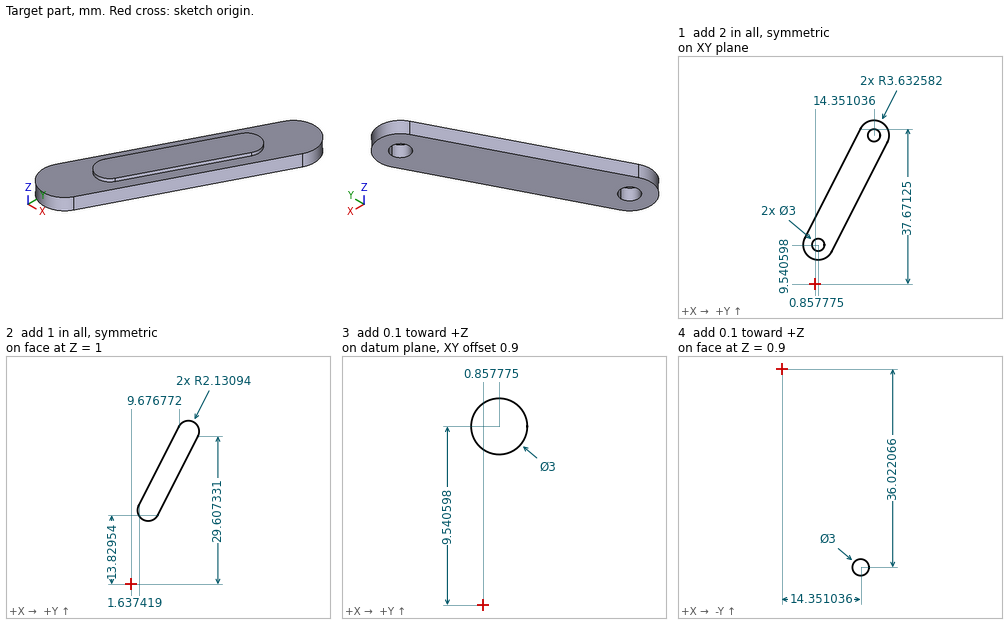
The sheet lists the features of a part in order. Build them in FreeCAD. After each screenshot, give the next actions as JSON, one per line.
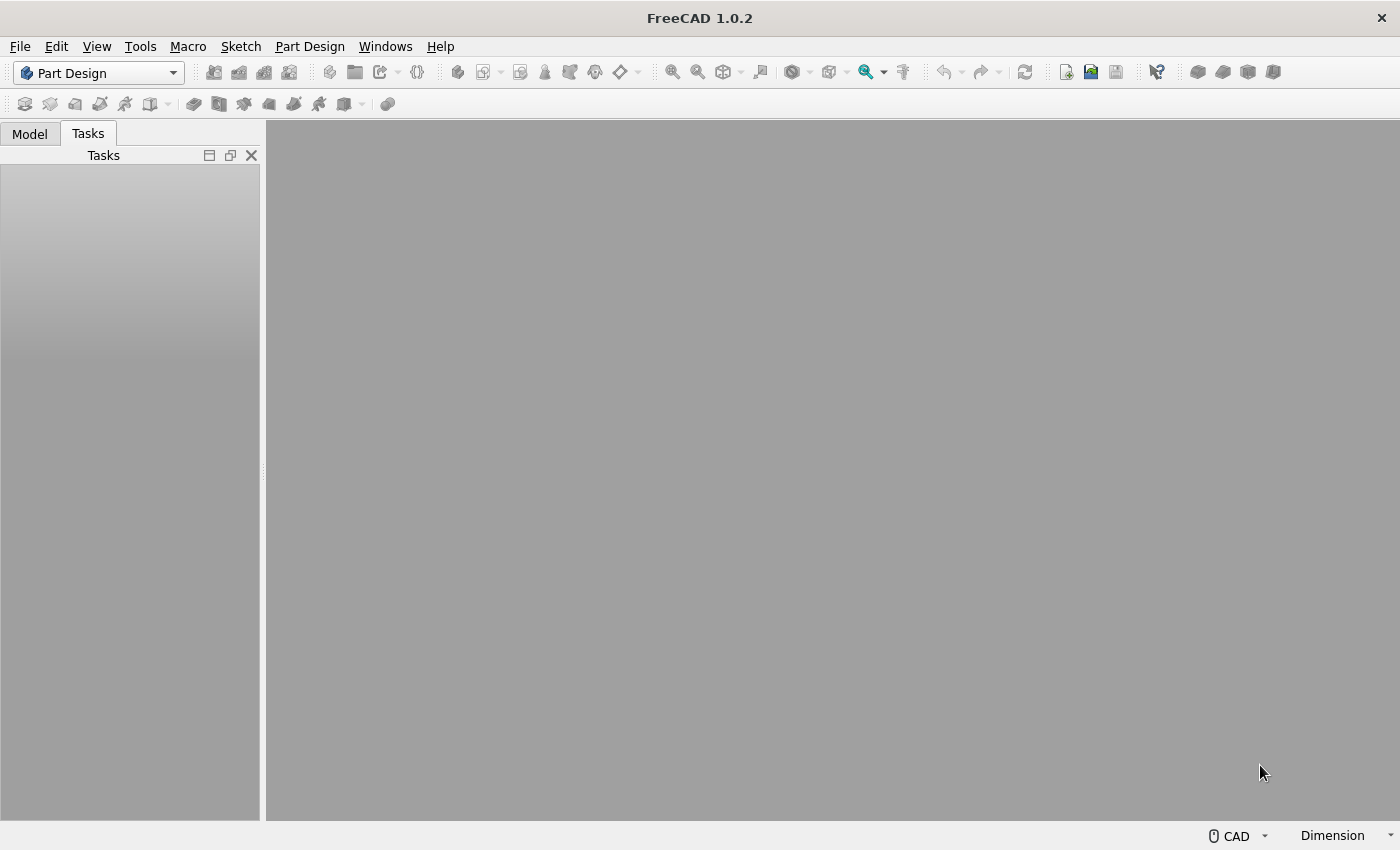
{"action": "left_click", "coordinate": [1066, 72]}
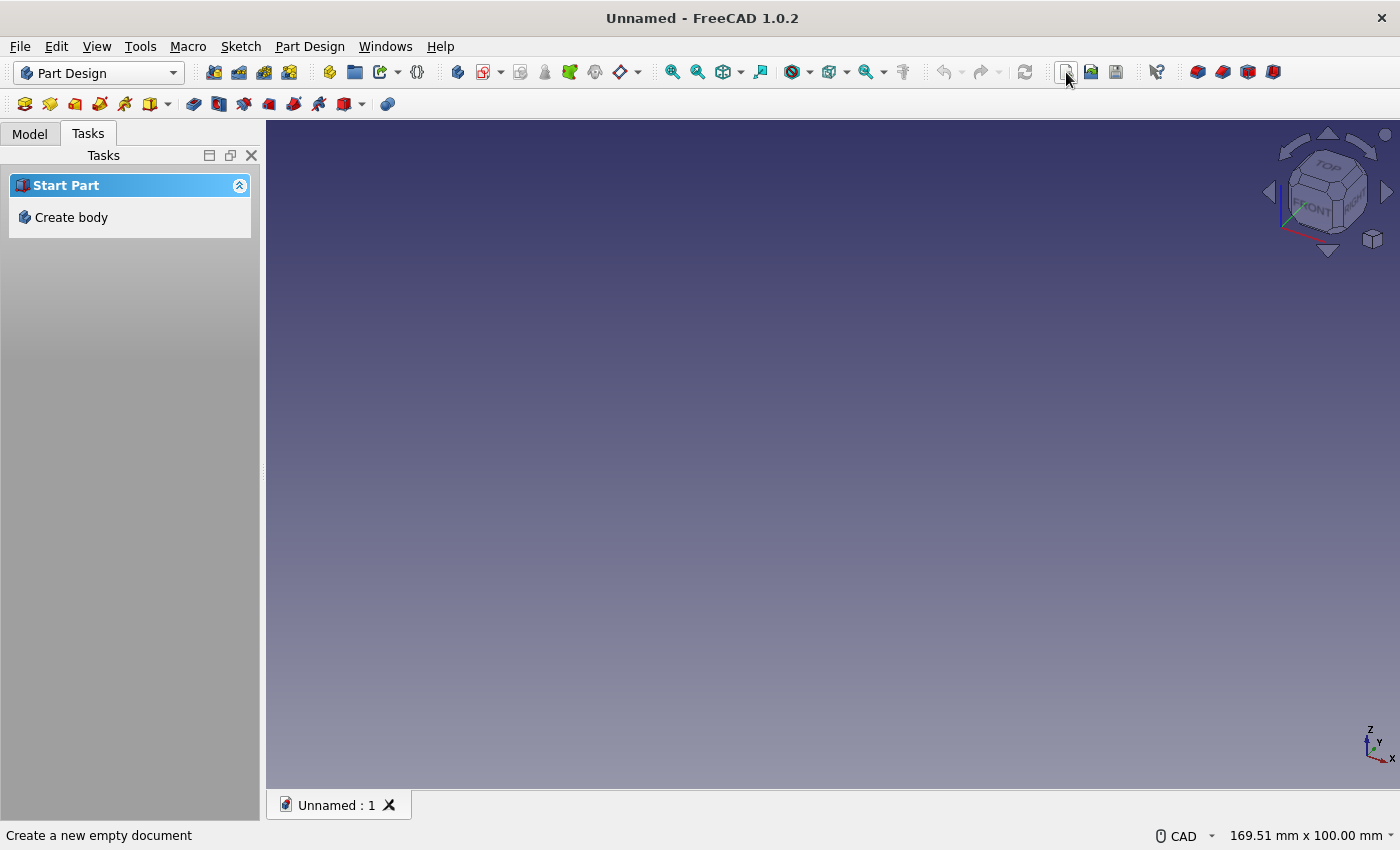
{"action": "left_click", "coordinate": [482, 72]}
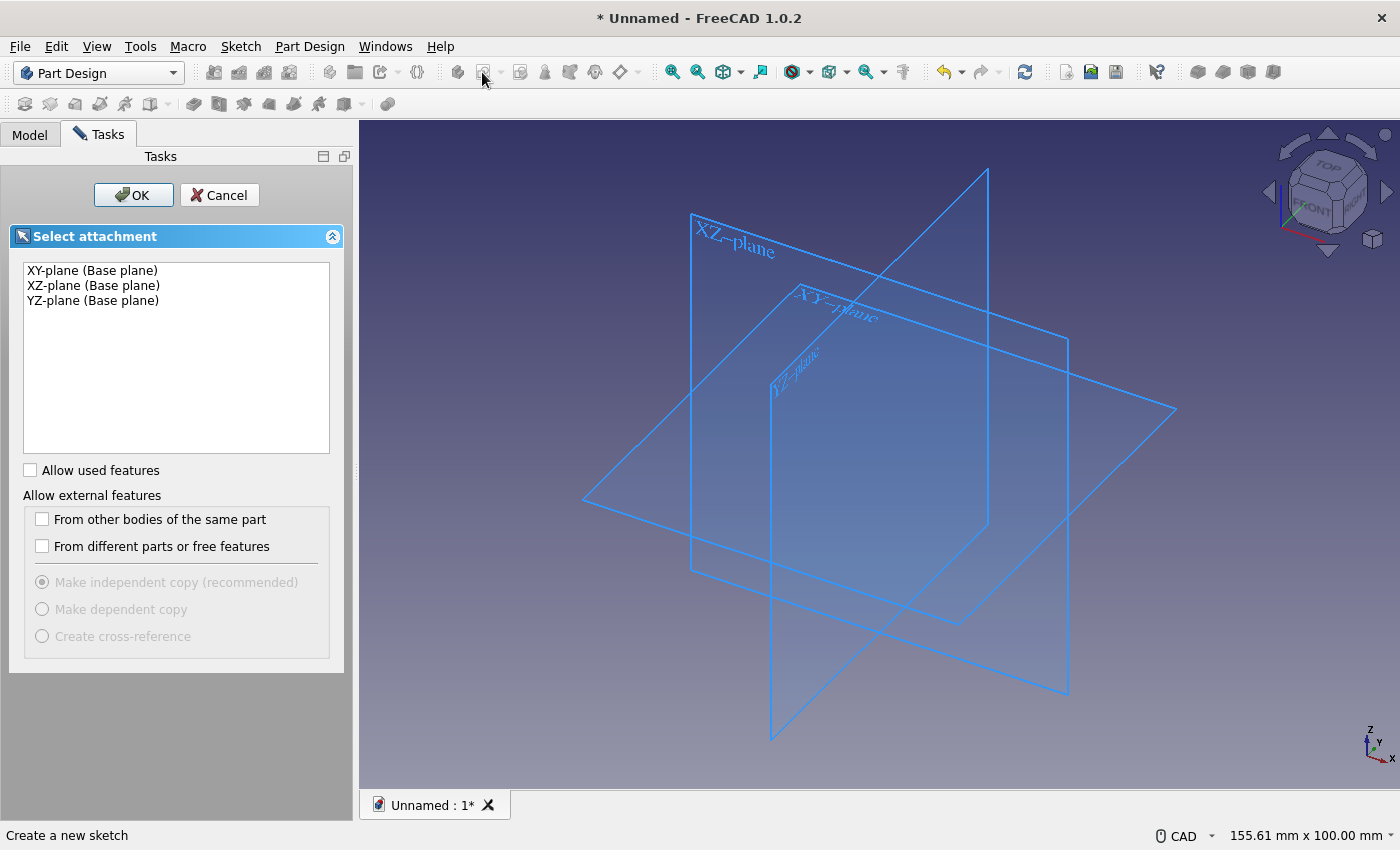
{"action": "left_click", "coordinate": [84, 270]}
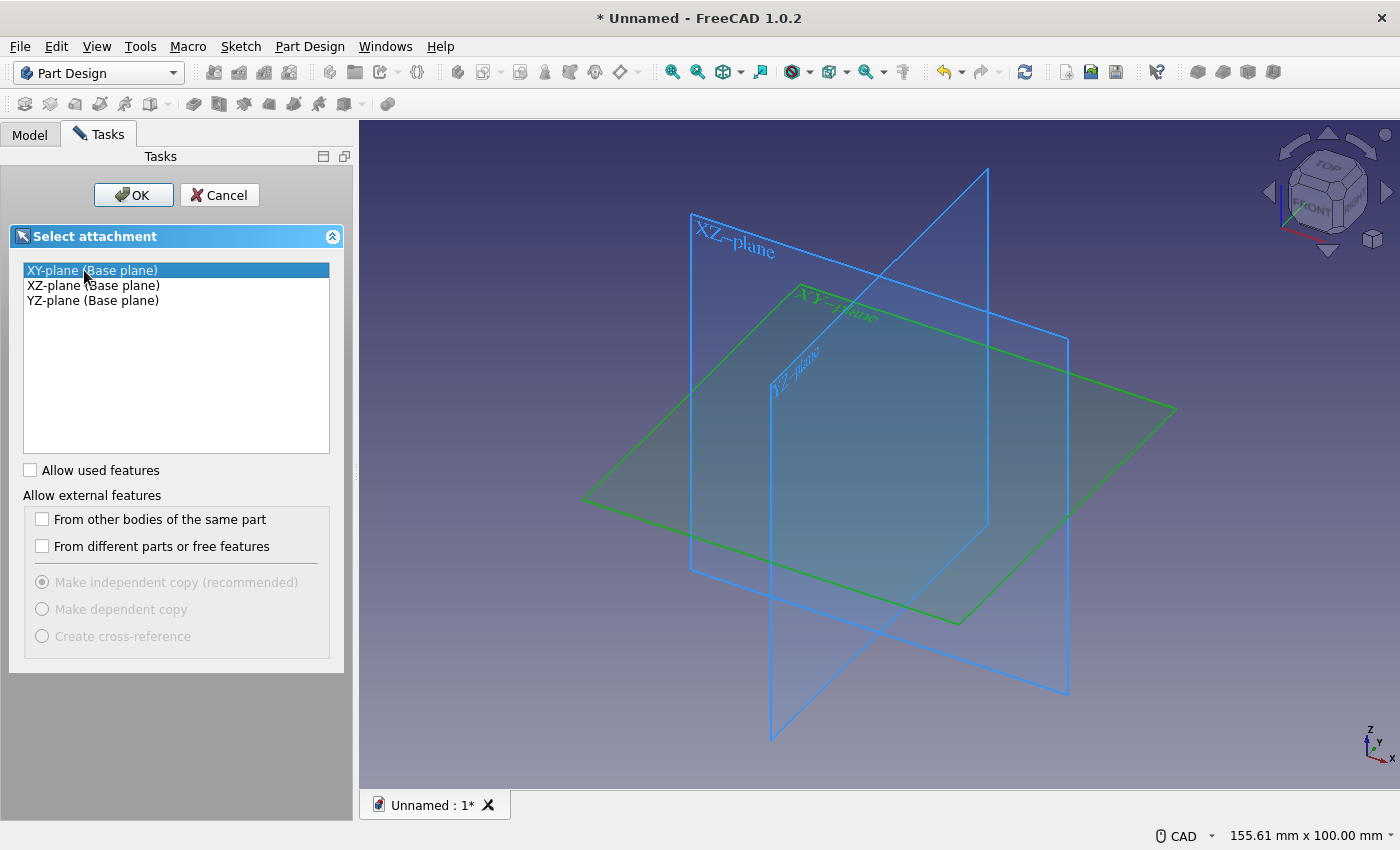
{"action": "left_click", "coordinate": [134, 195]}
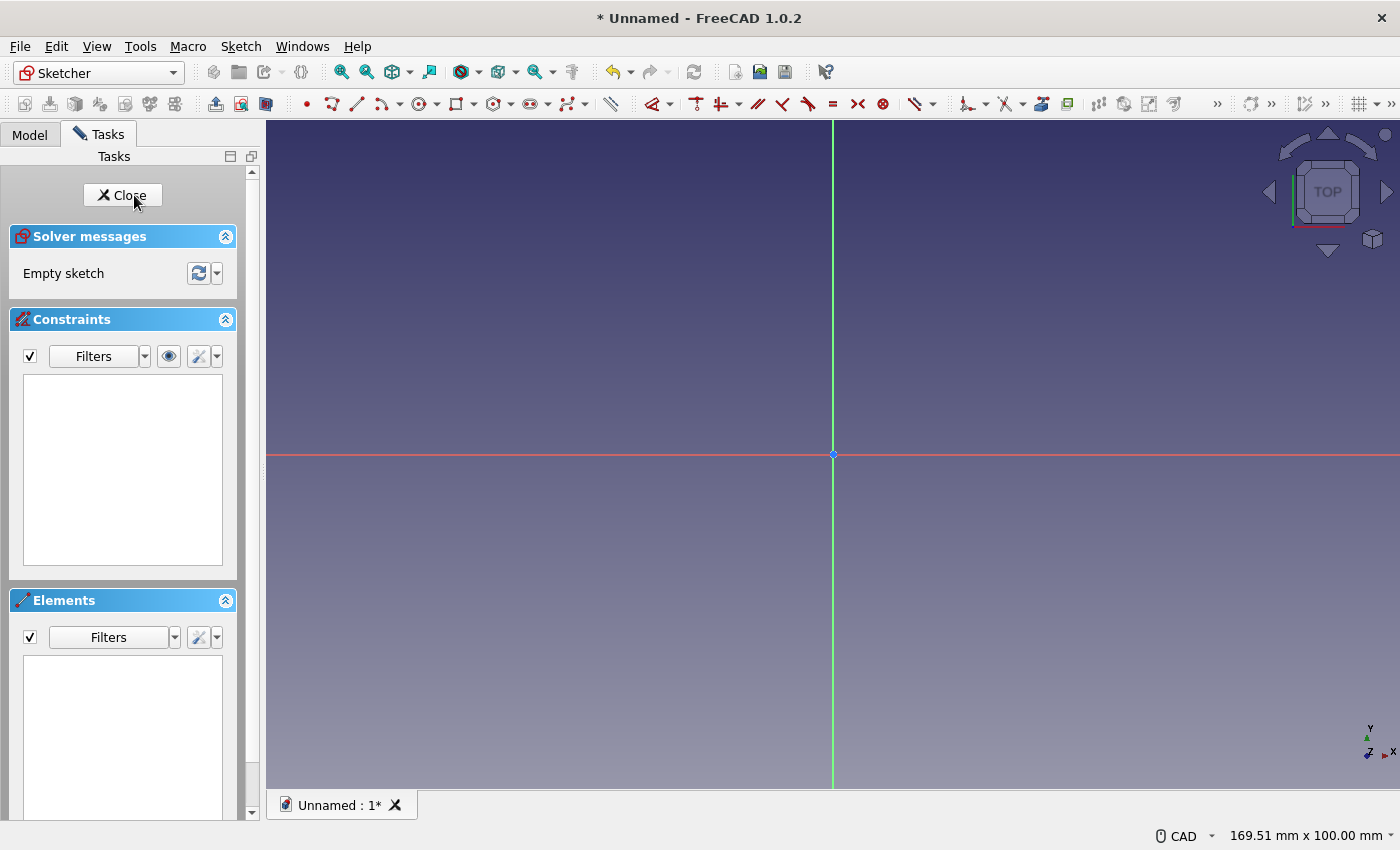
{"action": "scroll", "coordinate": [1127, 148], "scroll_direction": "up", "scroll_amount": 2}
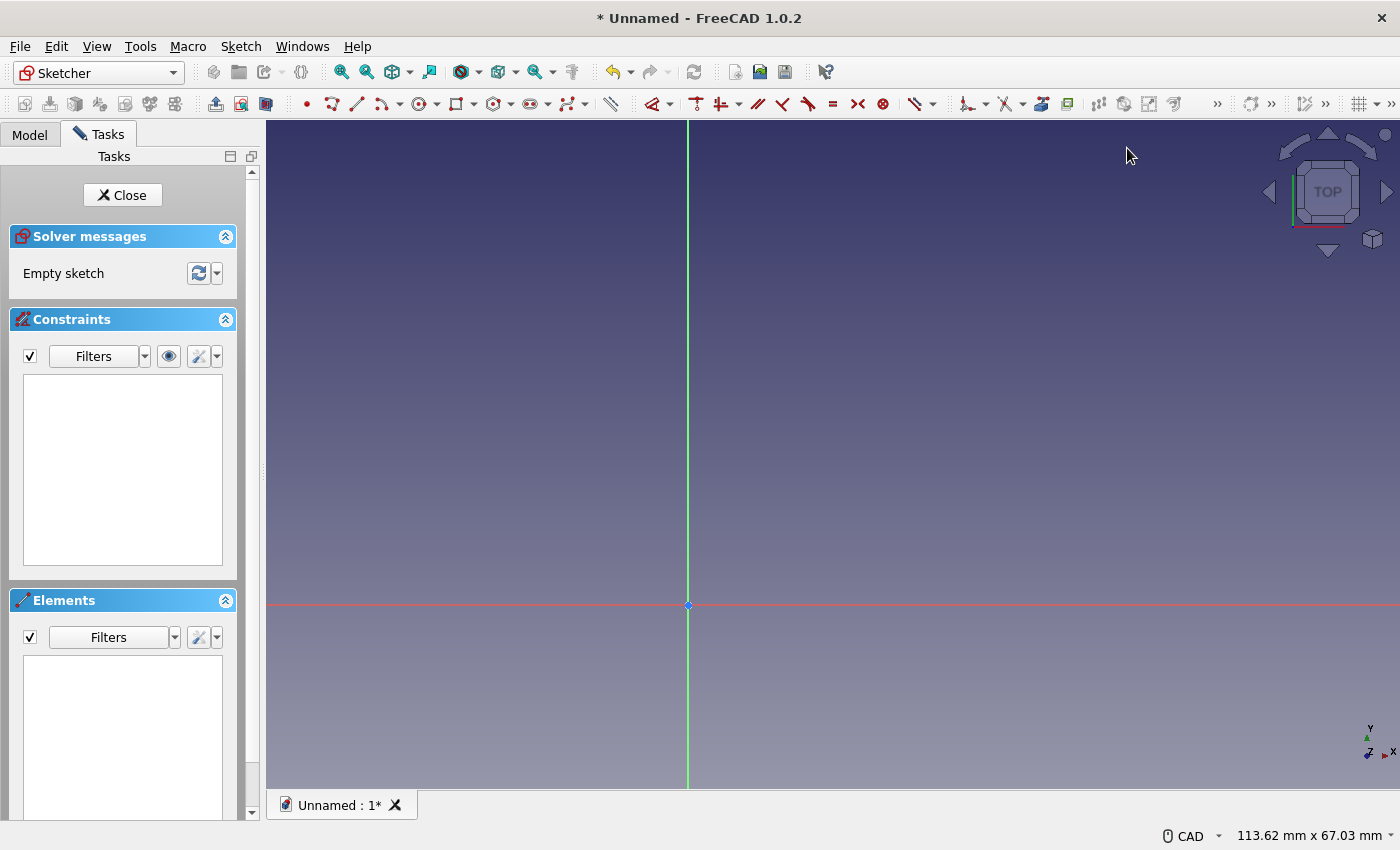
{"action": "key", "text": "g s"}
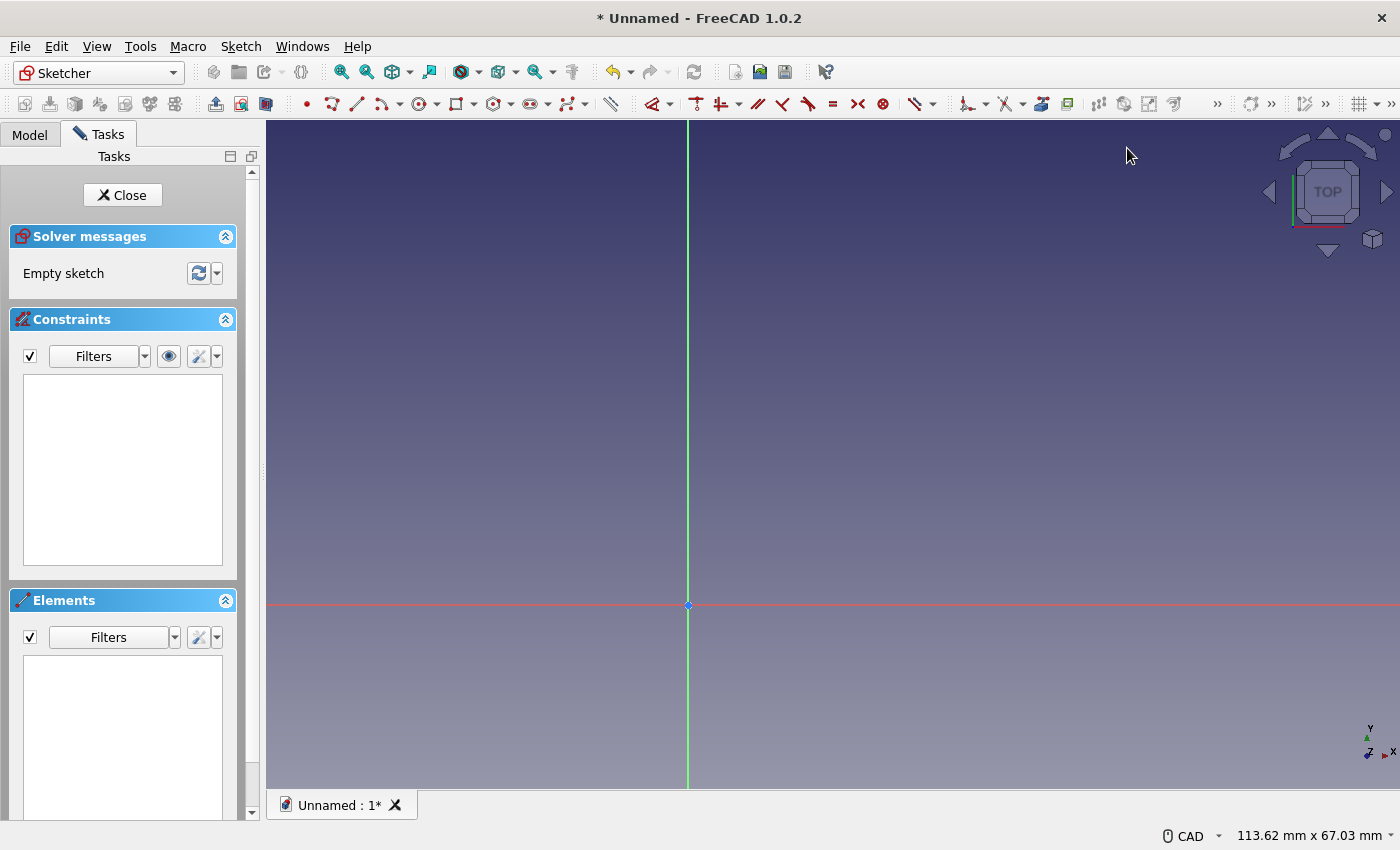
{"action": "scroll", "coordinate": [697, 510], "scroll_direction": "up", "scroll_amount": 4}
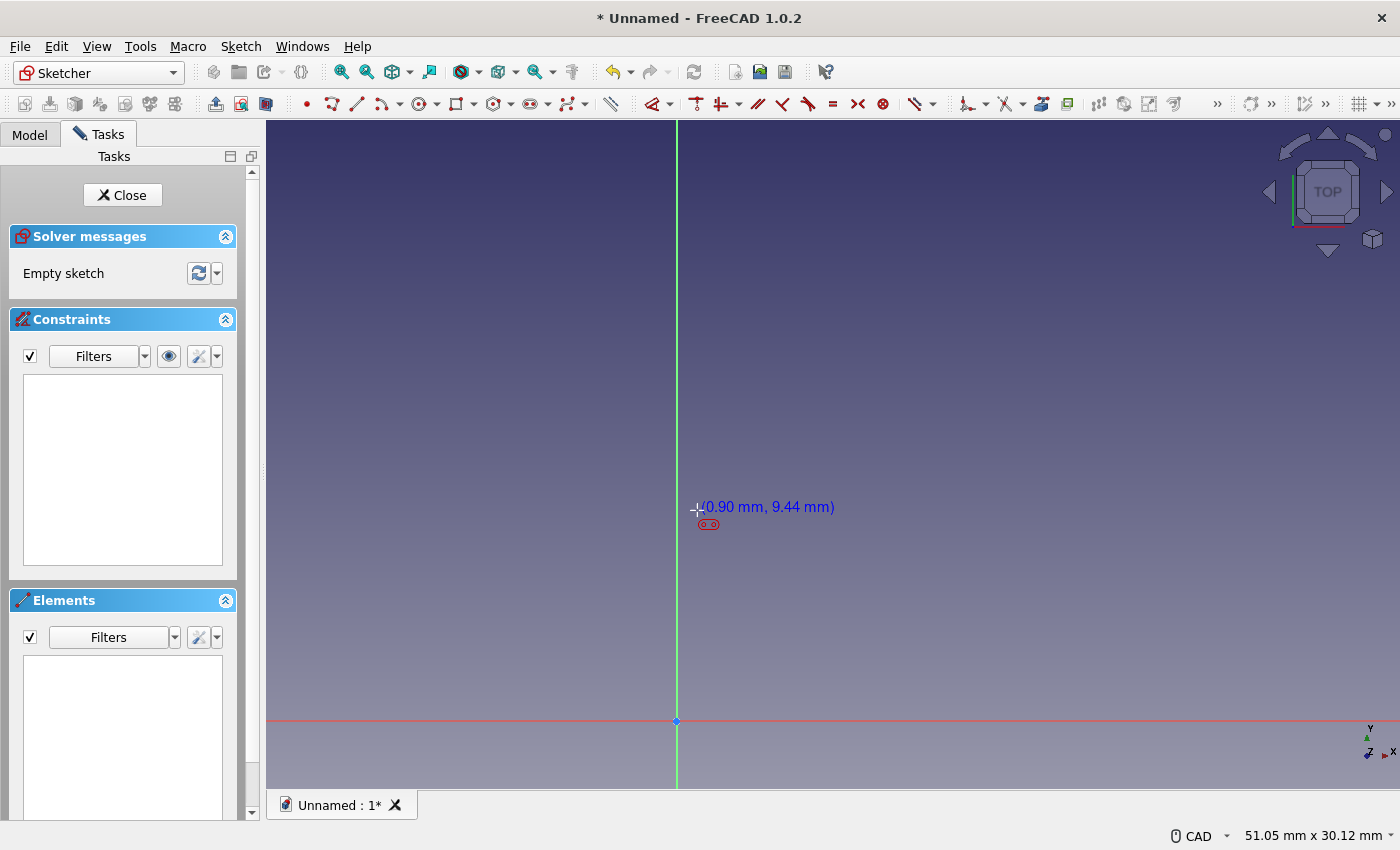
{"action": "left_click", "coordinate": [696, 509]}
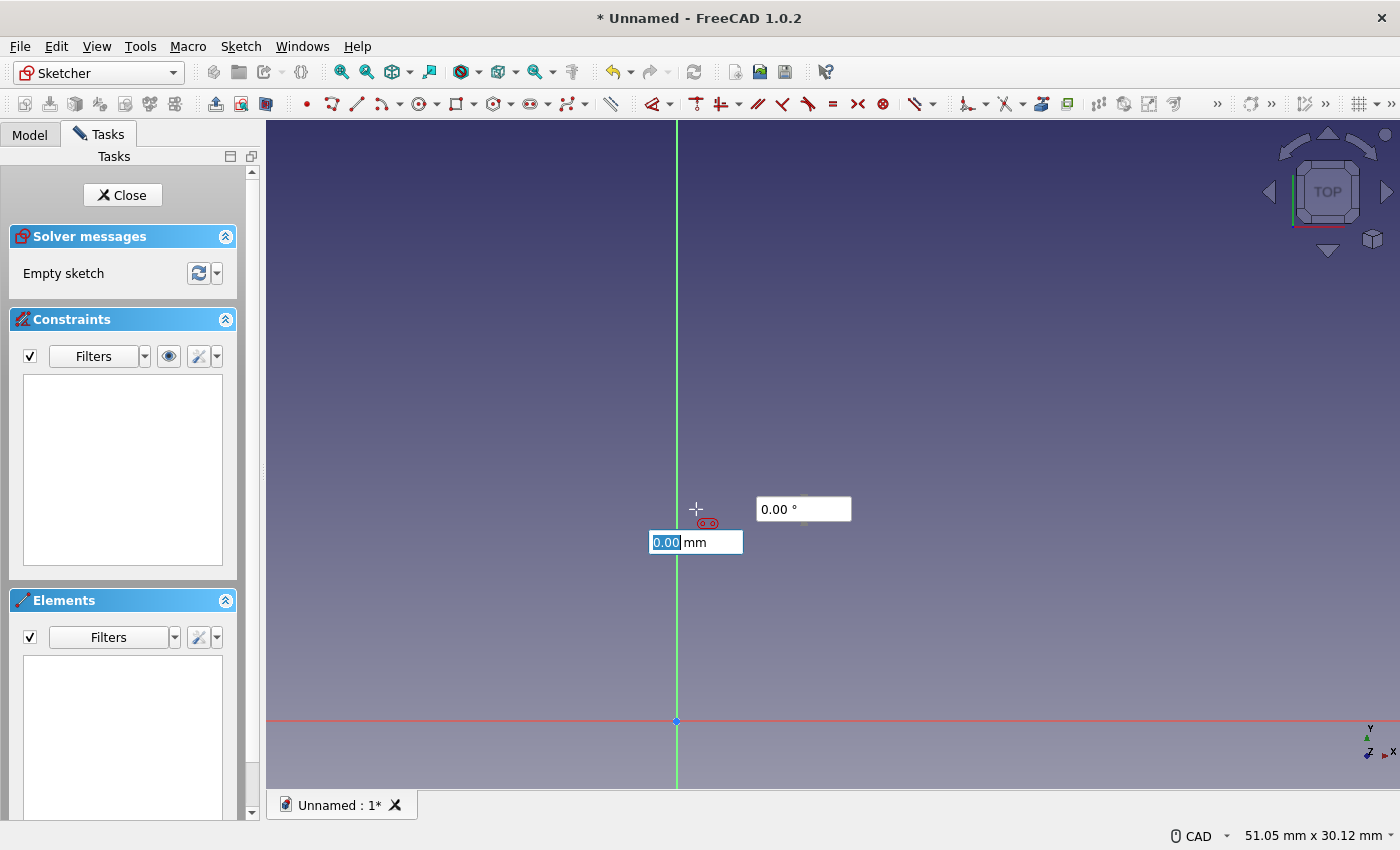
{"action": "scroll", "coordinate": [698, 593], "scroll_direction": "down", "scroll_amount": 4}